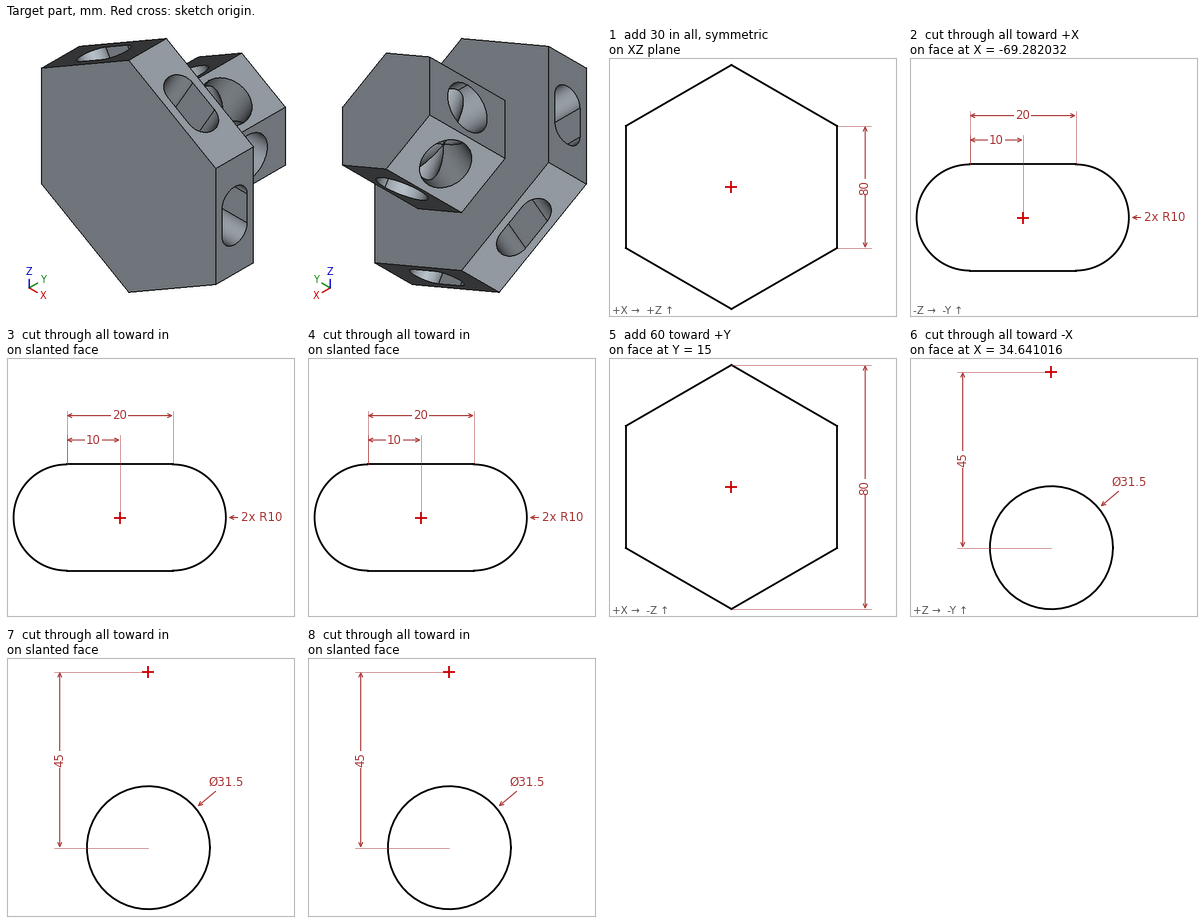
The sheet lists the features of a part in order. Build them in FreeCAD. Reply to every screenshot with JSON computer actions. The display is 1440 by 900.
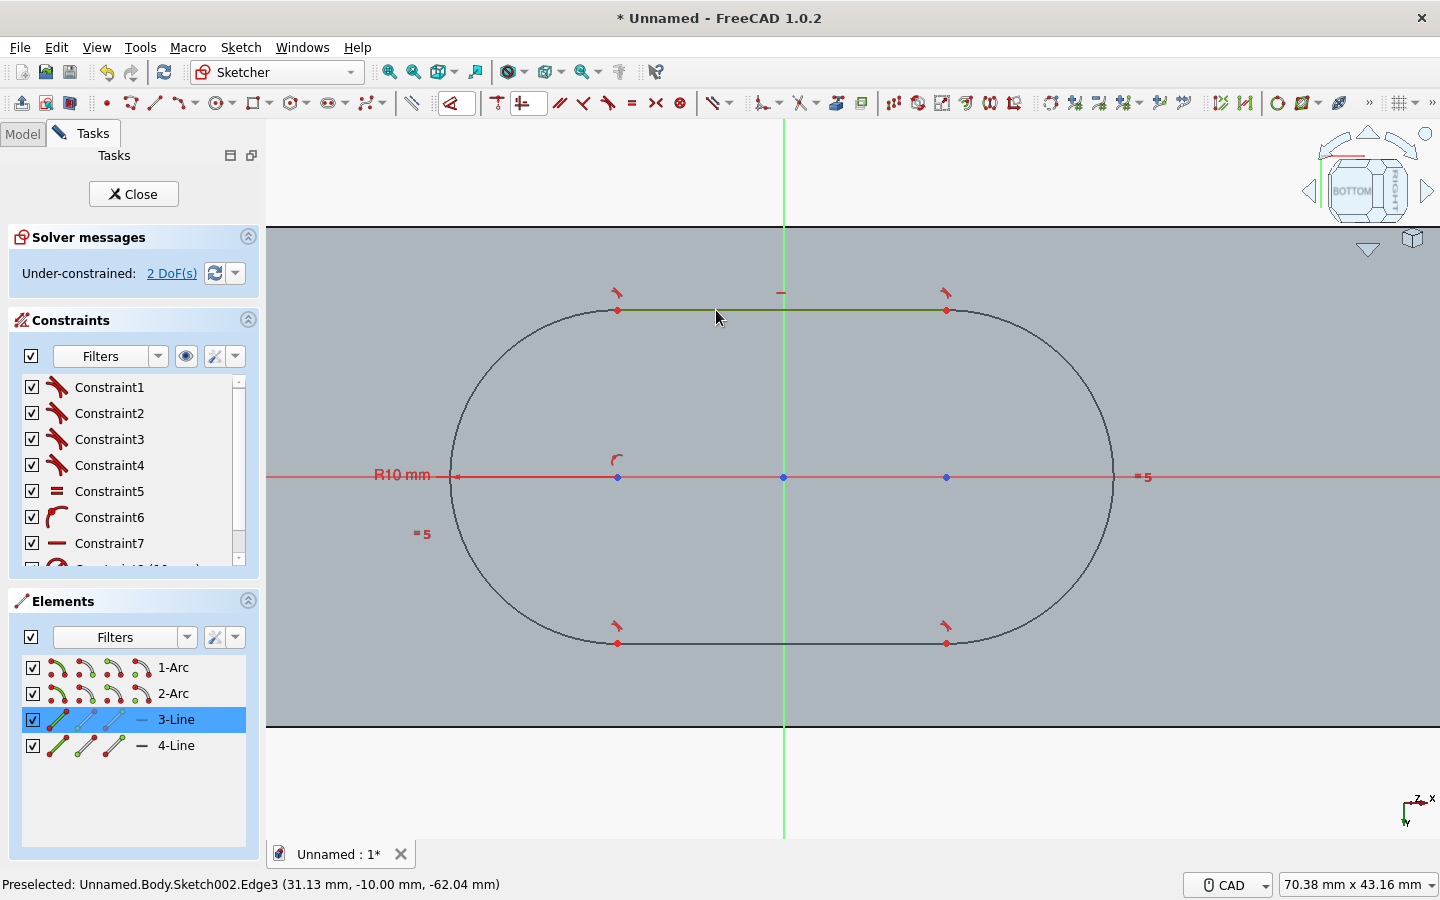
{"action": "key", "text": "l"}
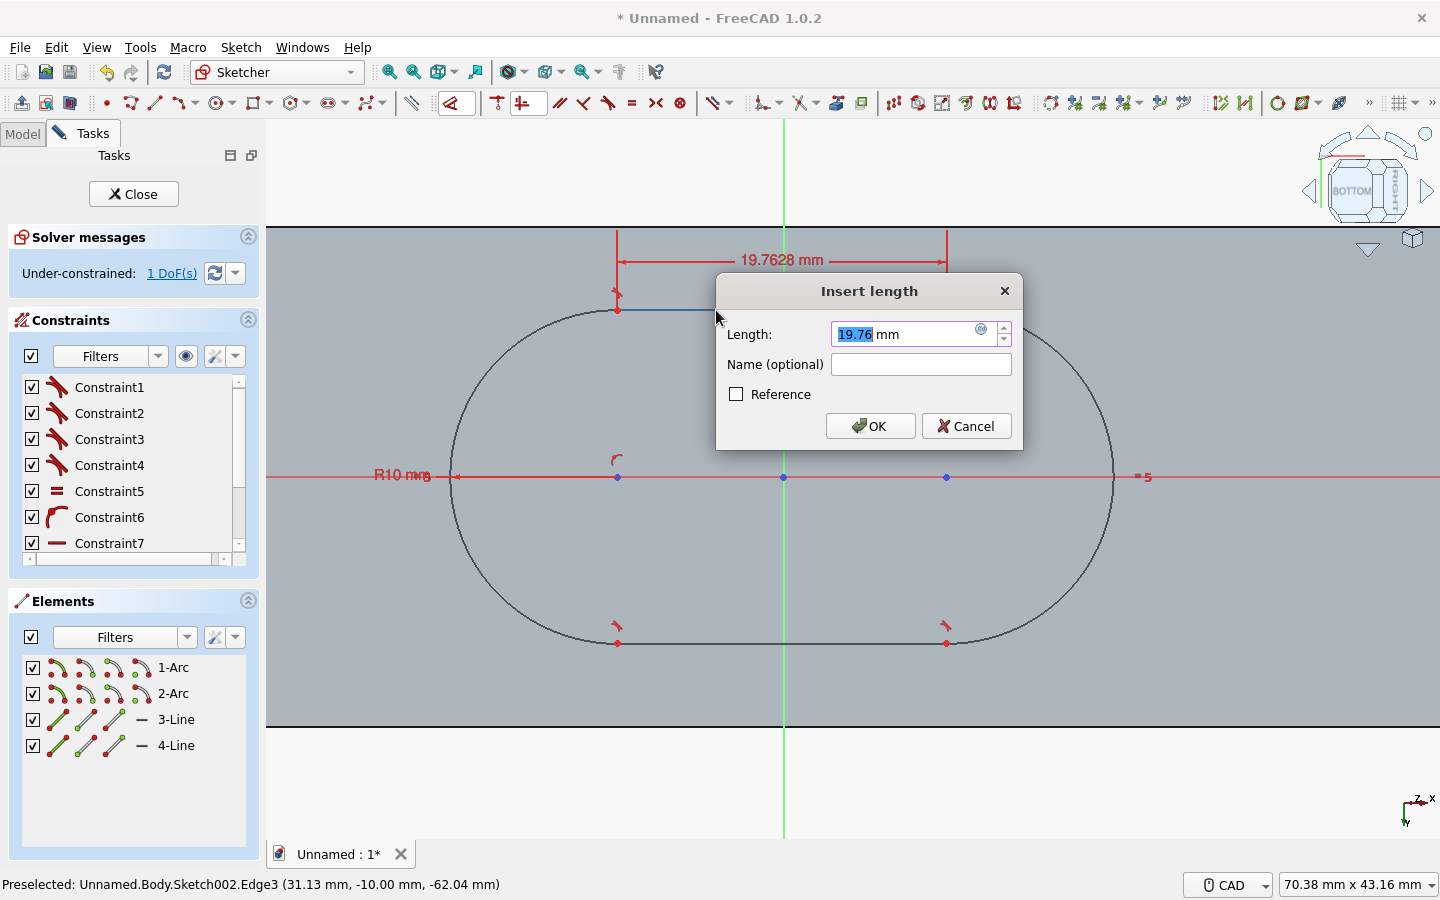
{"action": "type", "text": "20"}
{"action": "key", "text": "Return"}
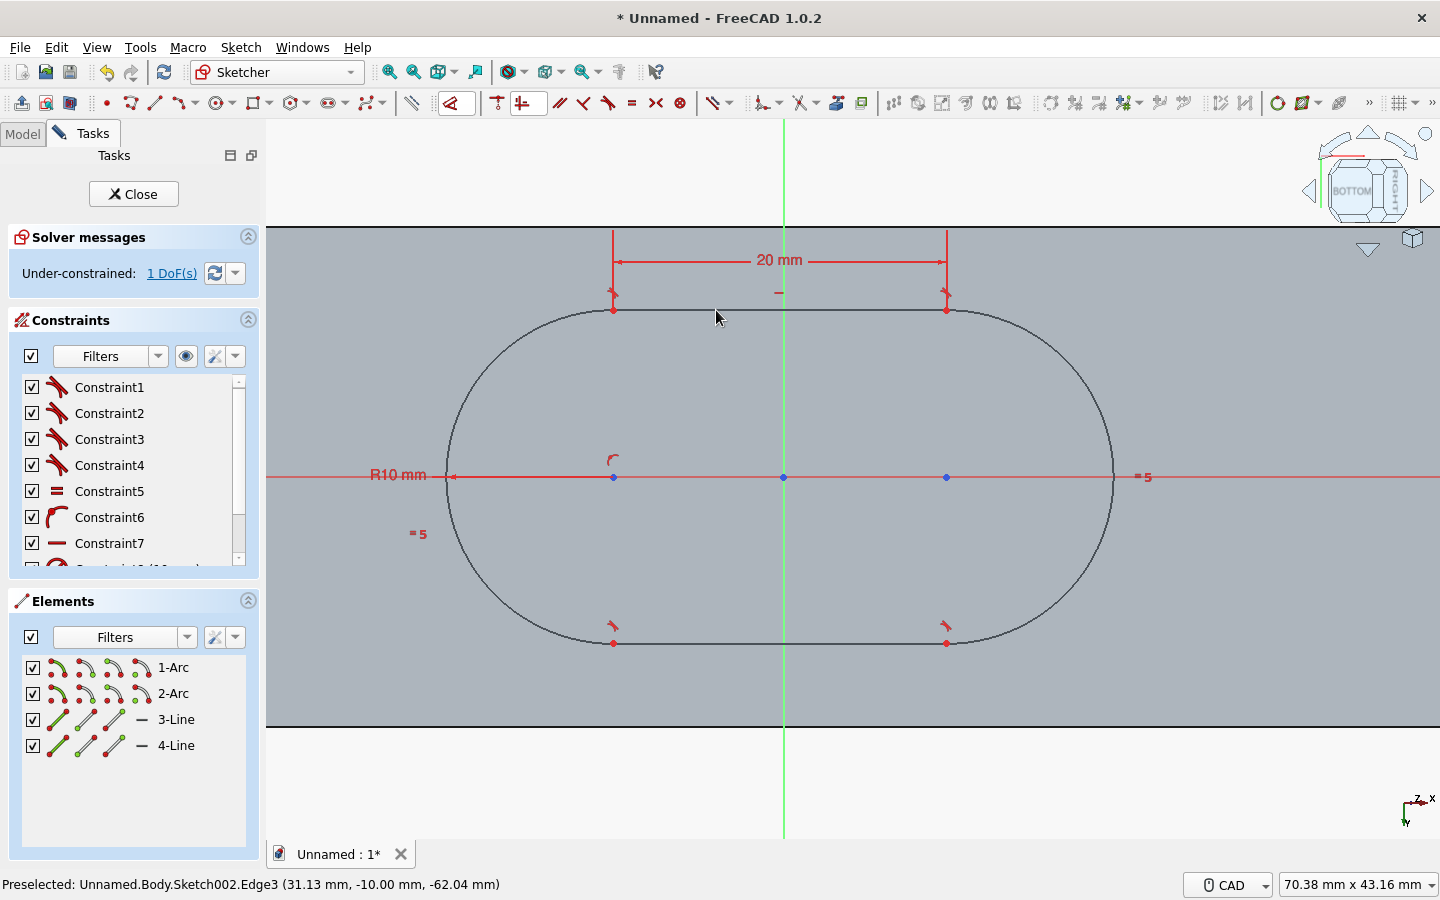
{"action": "left_click", "coordinate": [613, 310]}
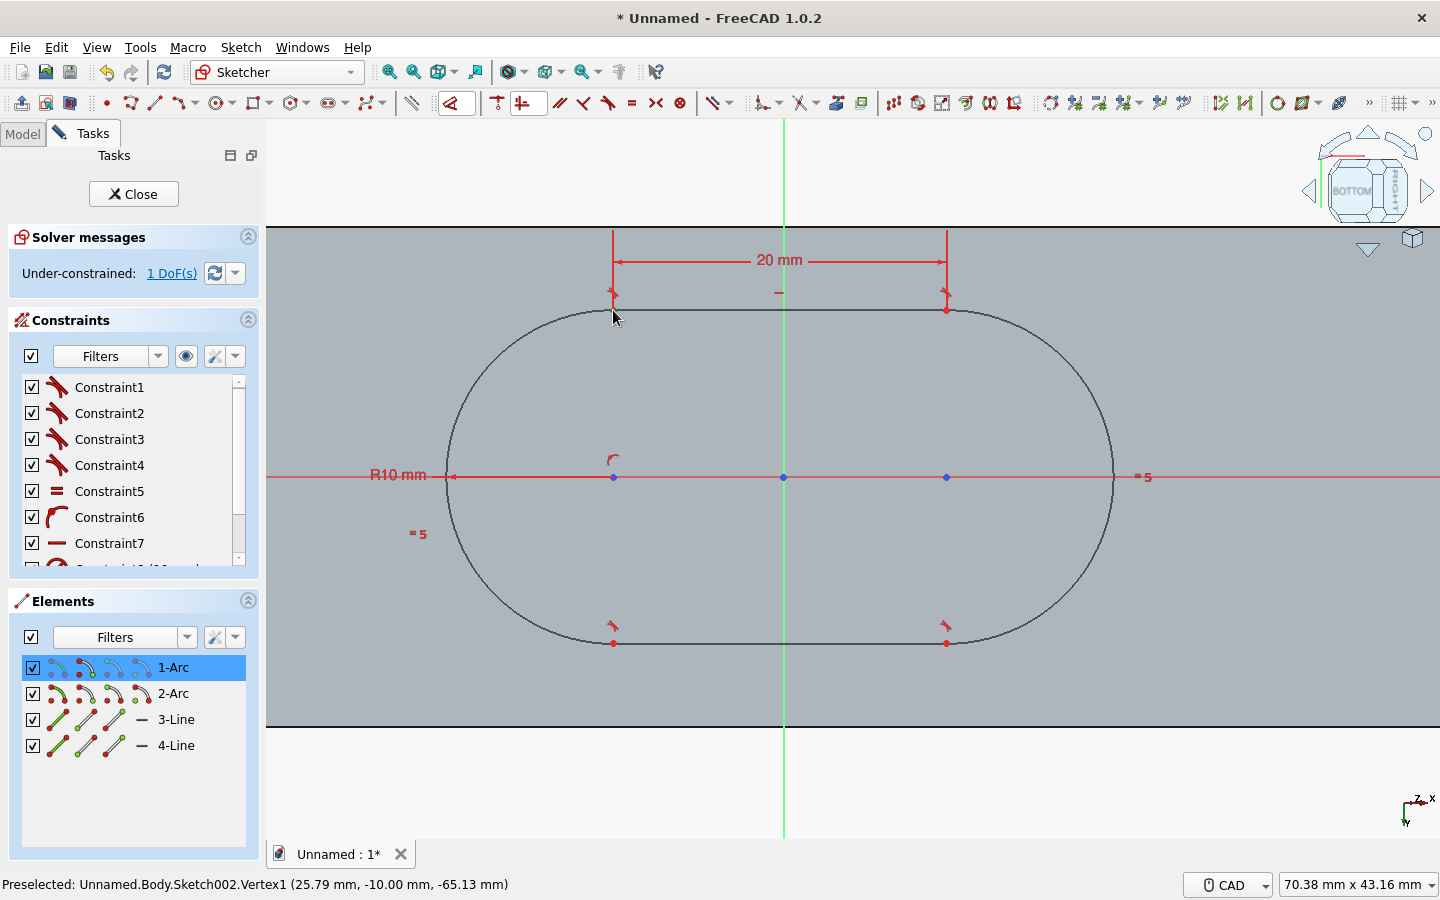
{"action": "left_click", "coordinate": [470, 104]}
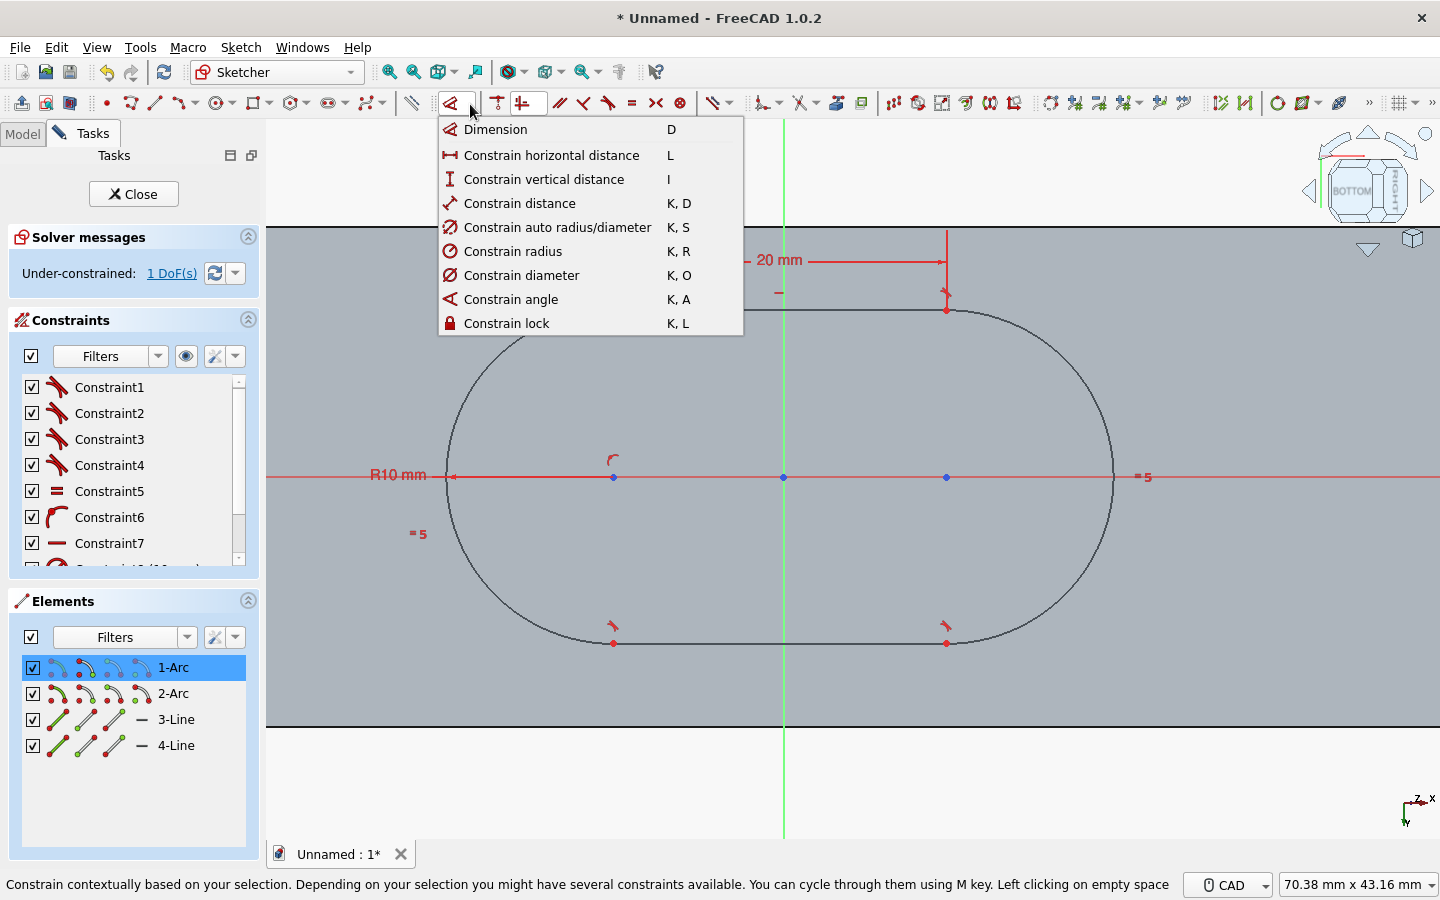
{"action": "left_click", "coordinate": [591, 155]}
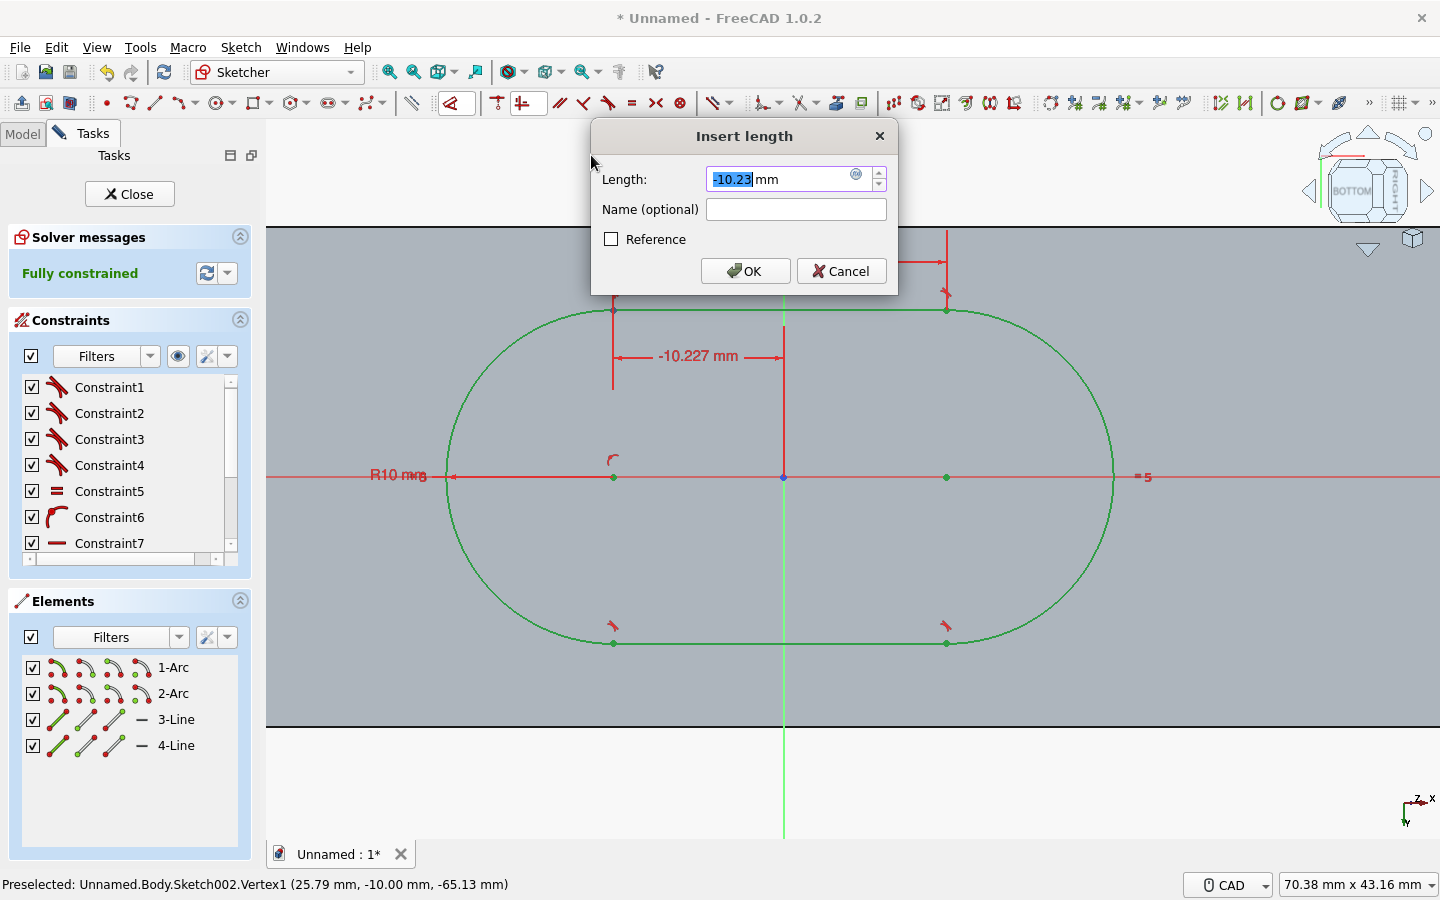
{"action": "type", "text": "-10"}
{"action": "key", "text": "Return"}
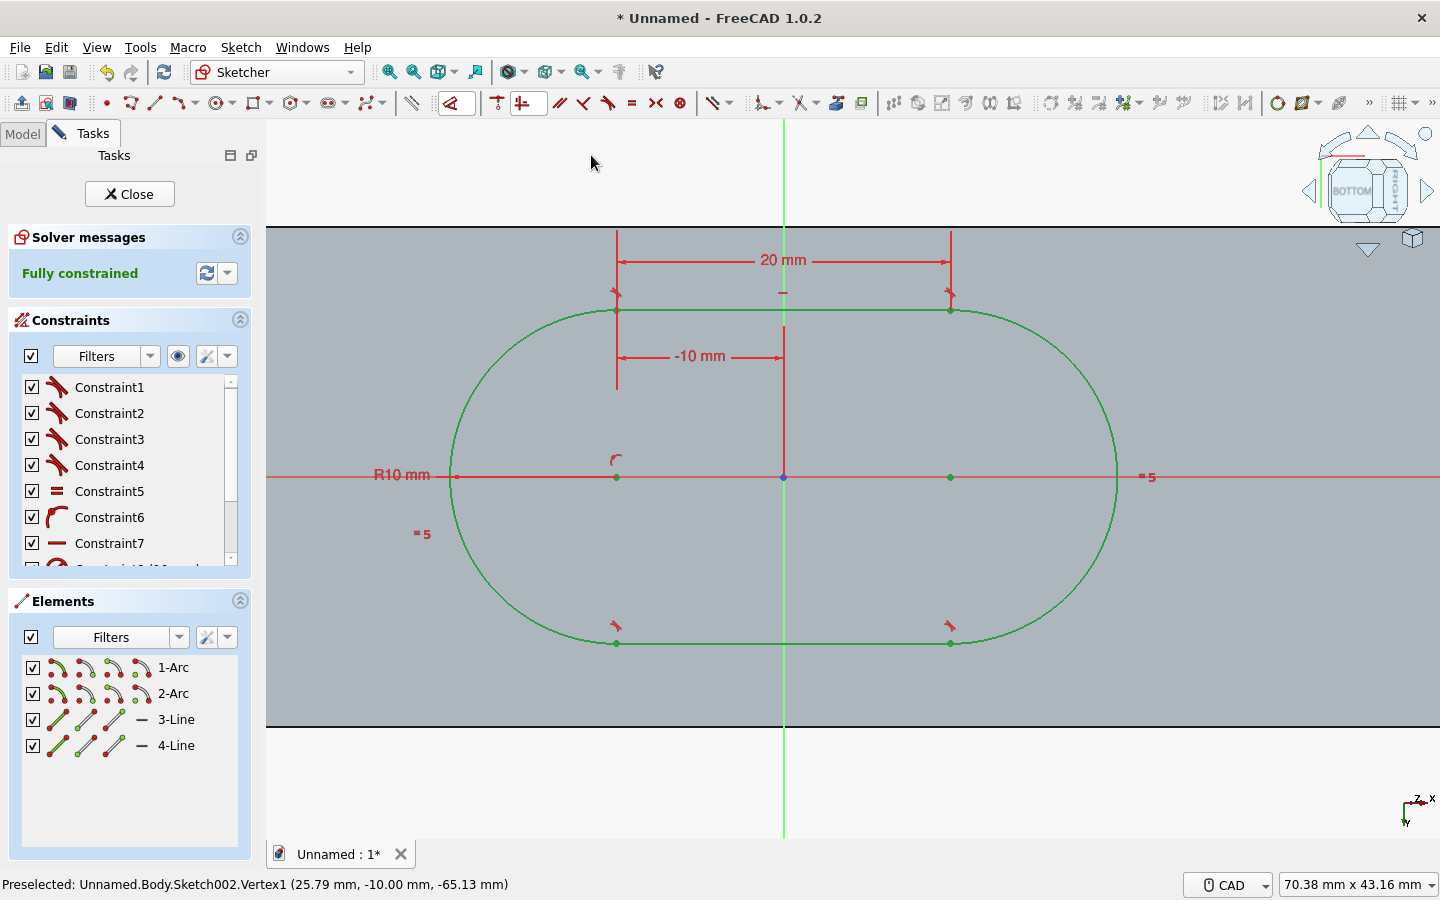
{"action": "left_click", "coordinate": [130, 194]}